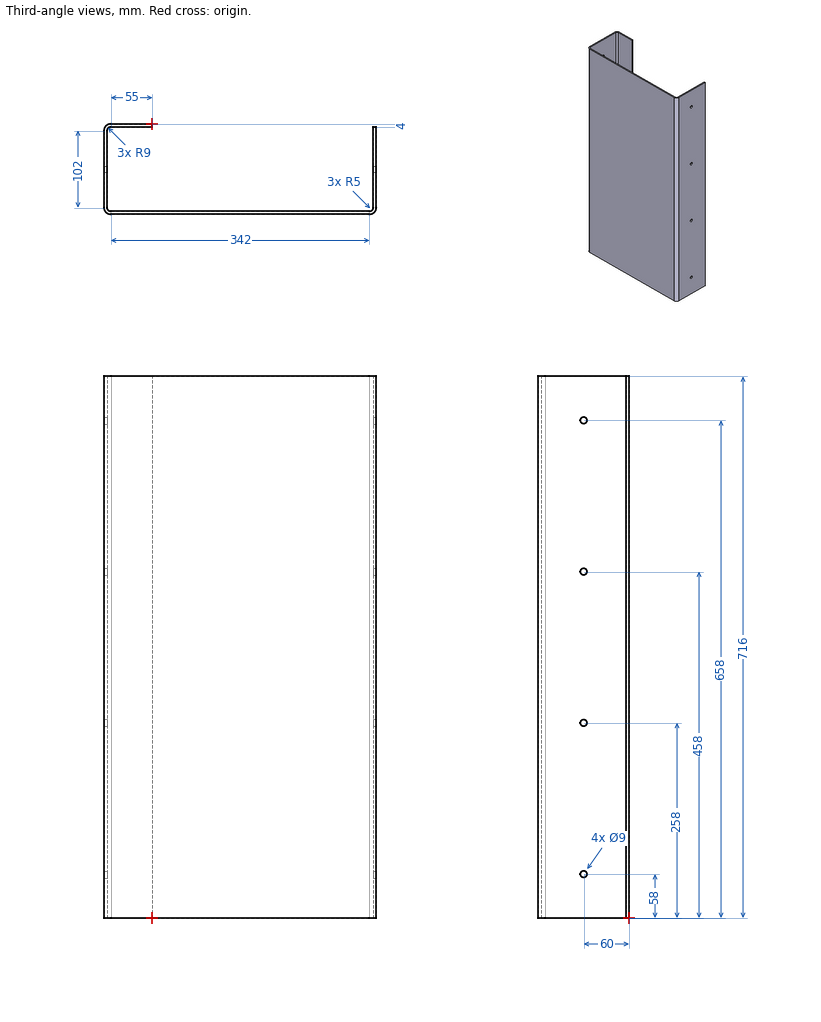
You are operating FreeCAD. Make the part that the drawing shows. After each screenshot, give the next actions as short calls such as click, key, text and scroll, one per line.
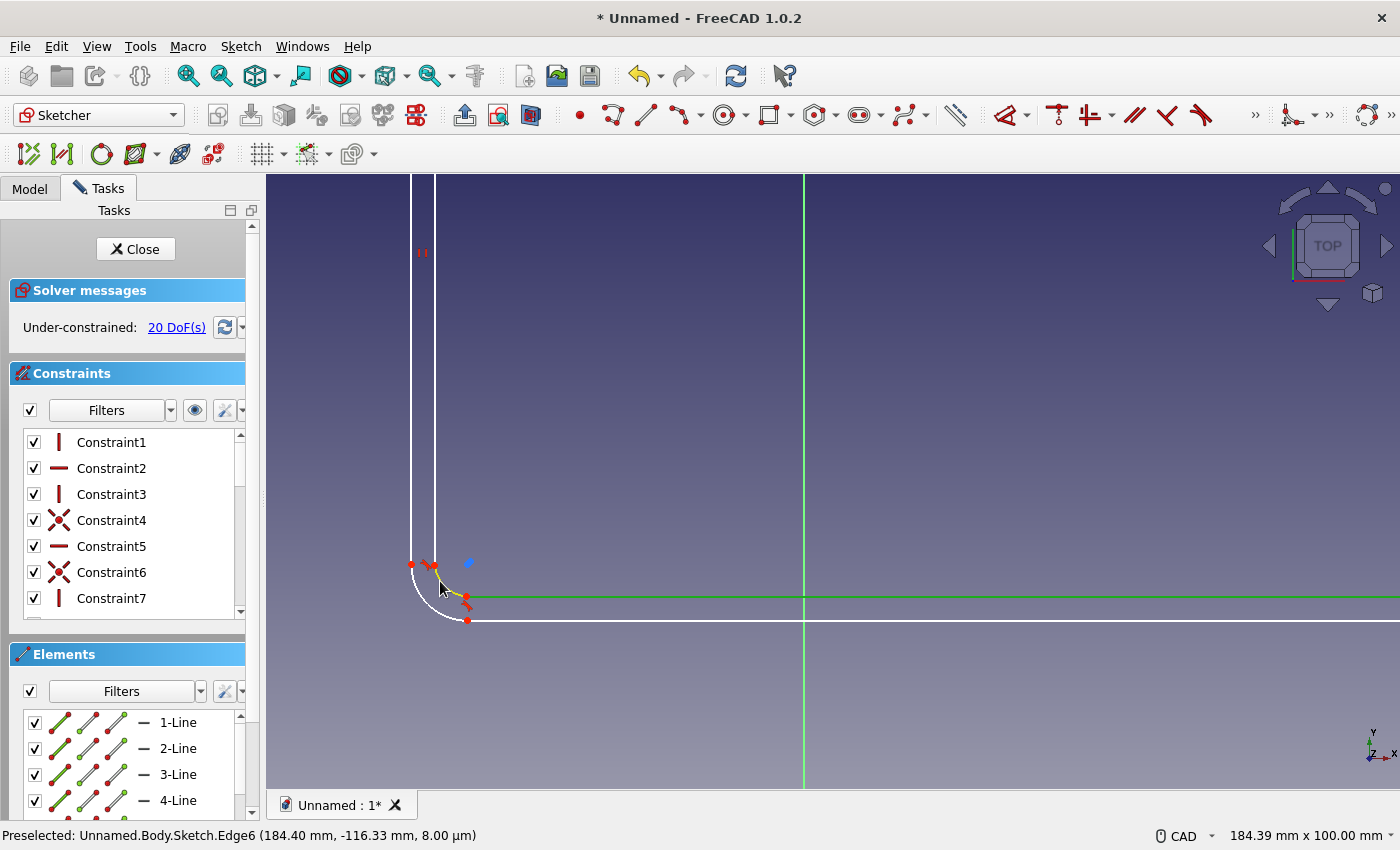
click(439, 579)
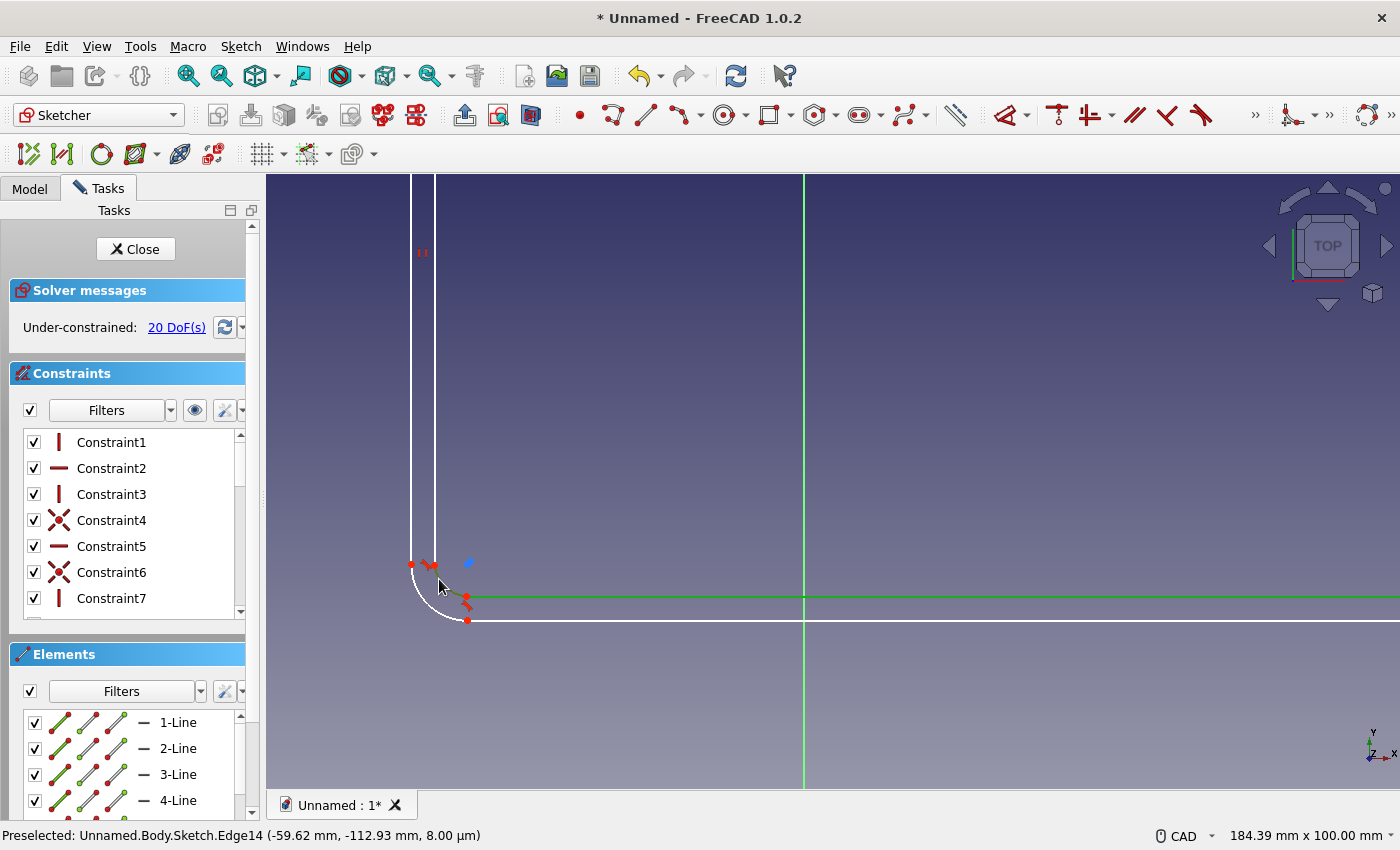
click(1201, 116)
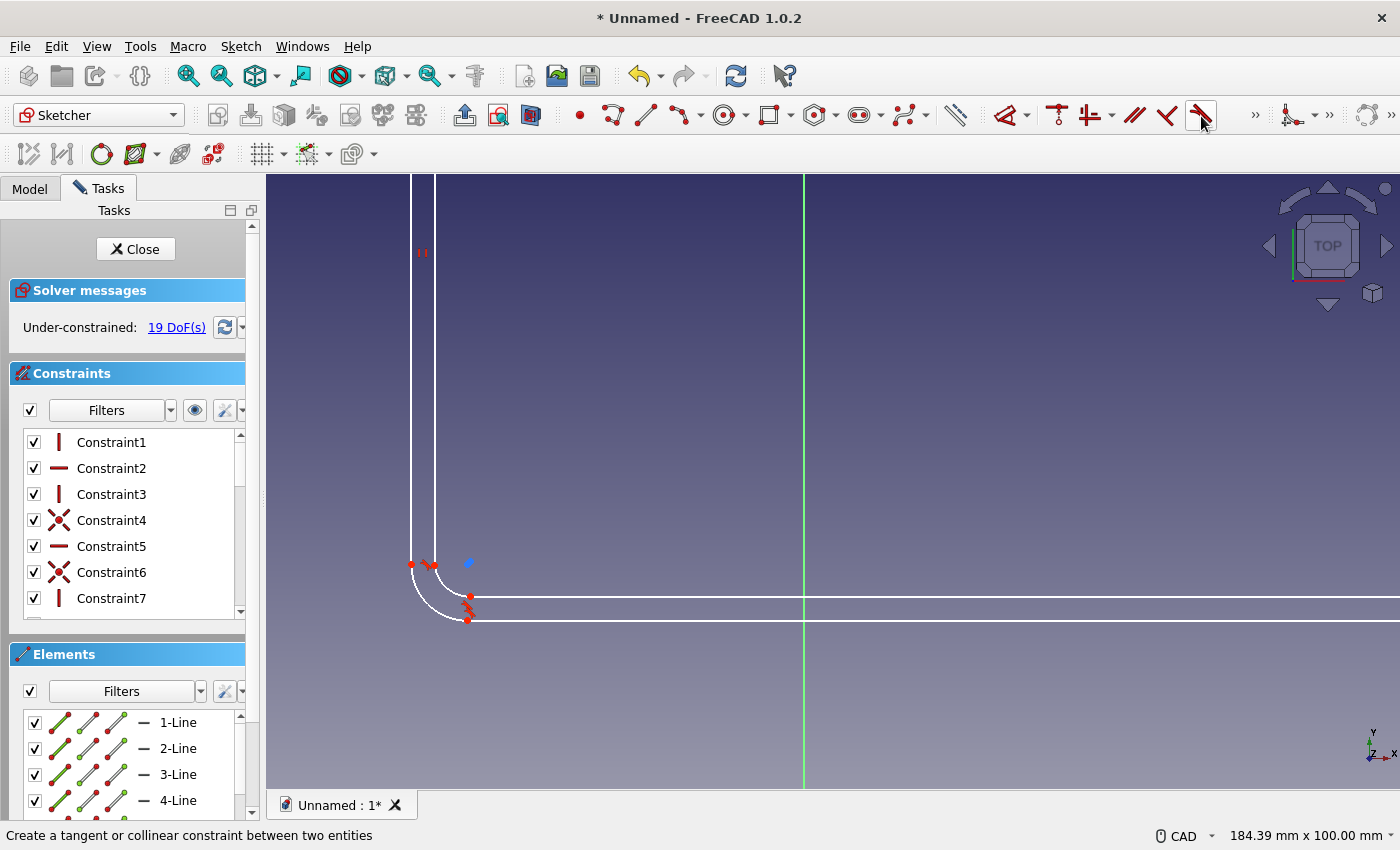
click(435, 378)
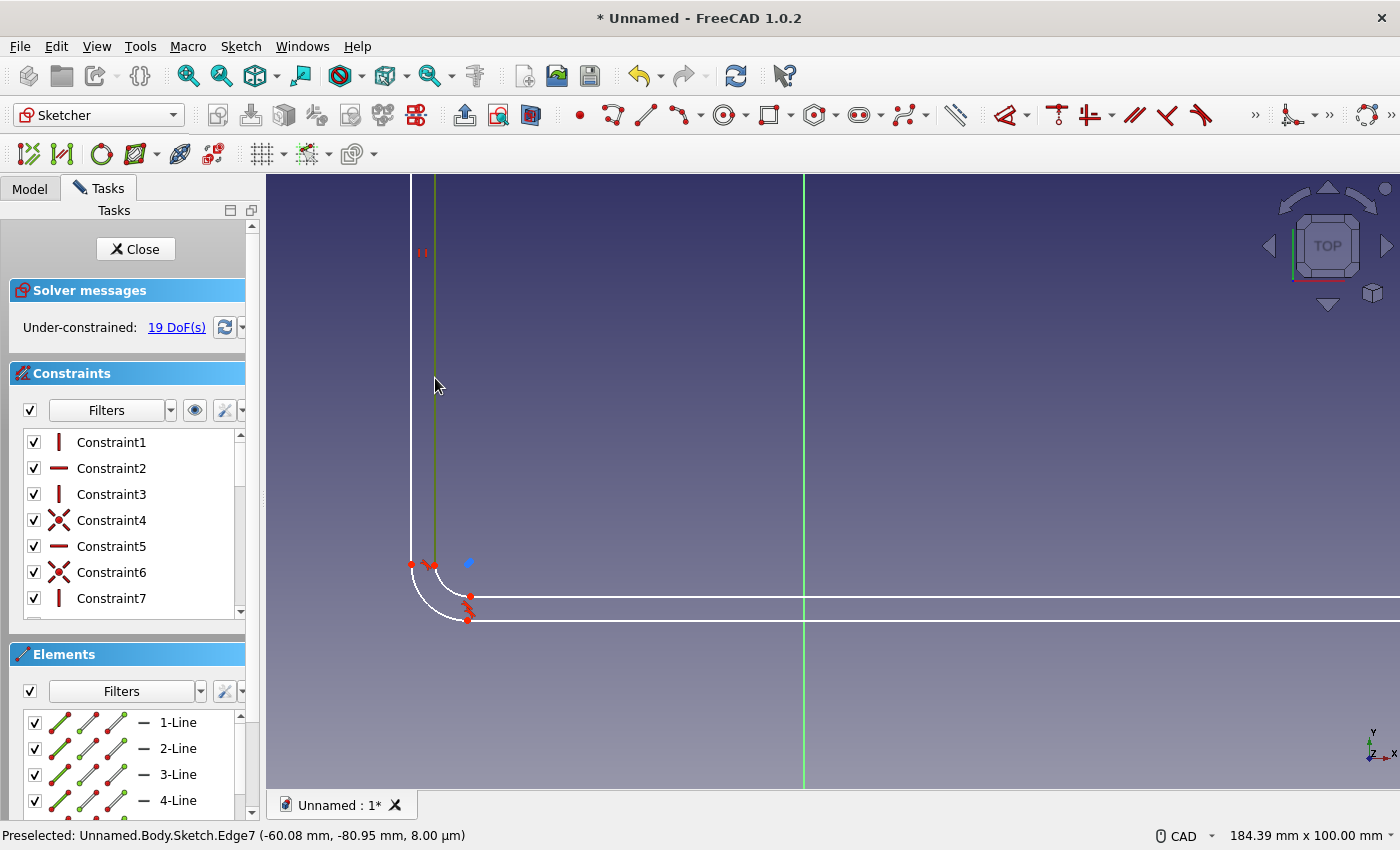
click(440, 580)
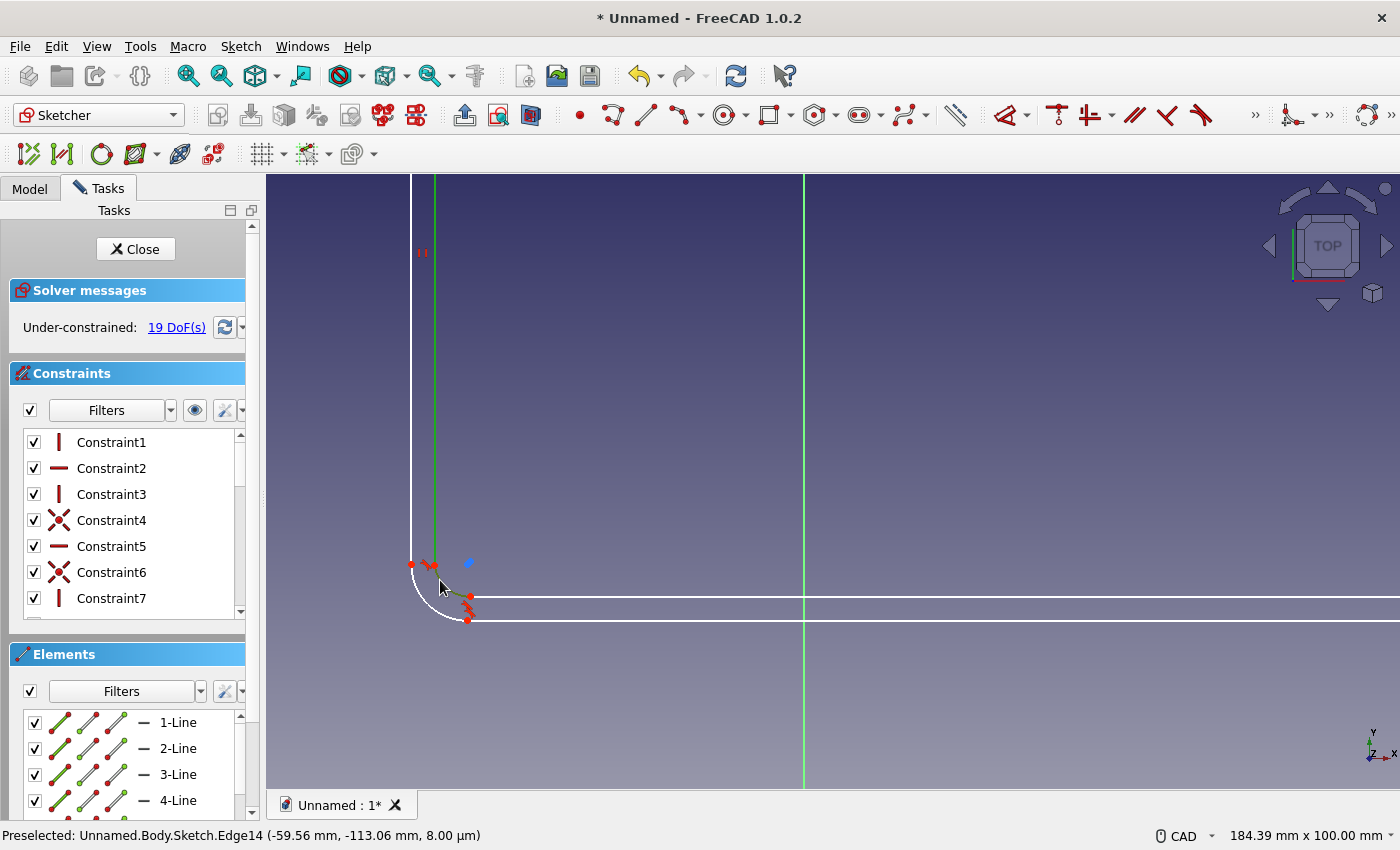
click(1201, 116)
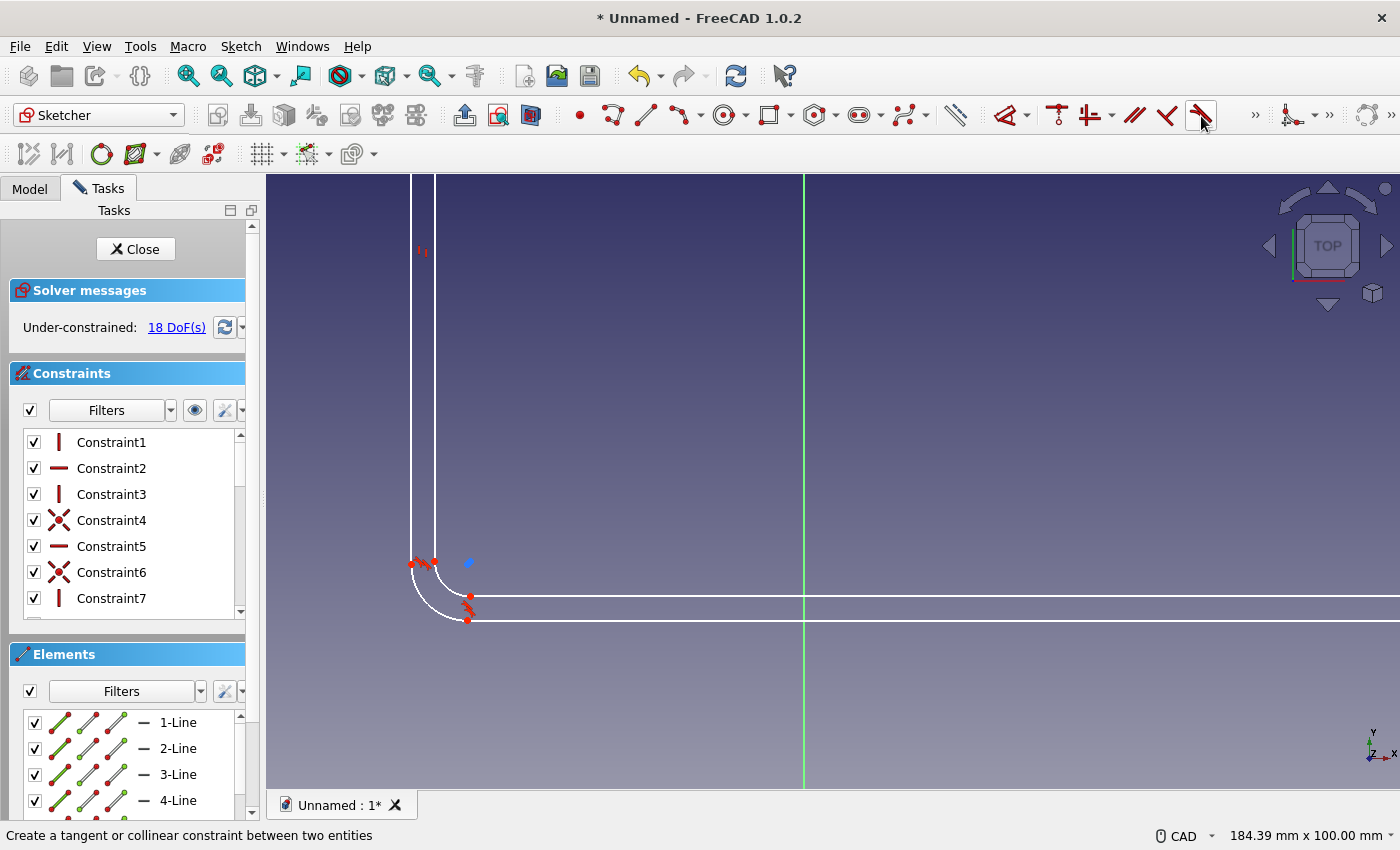
click(435, 374)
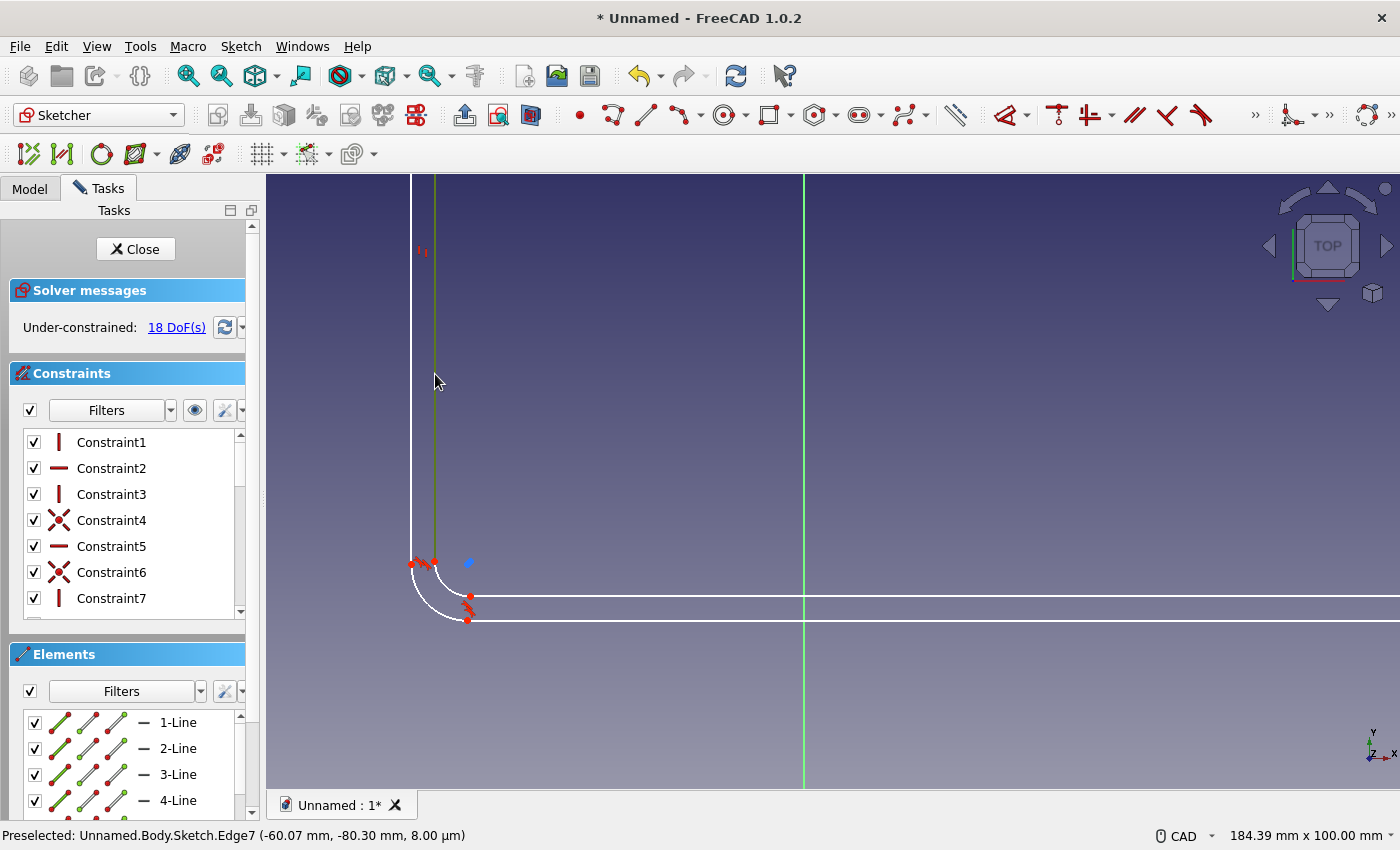
scroll(440, 581, down, 6)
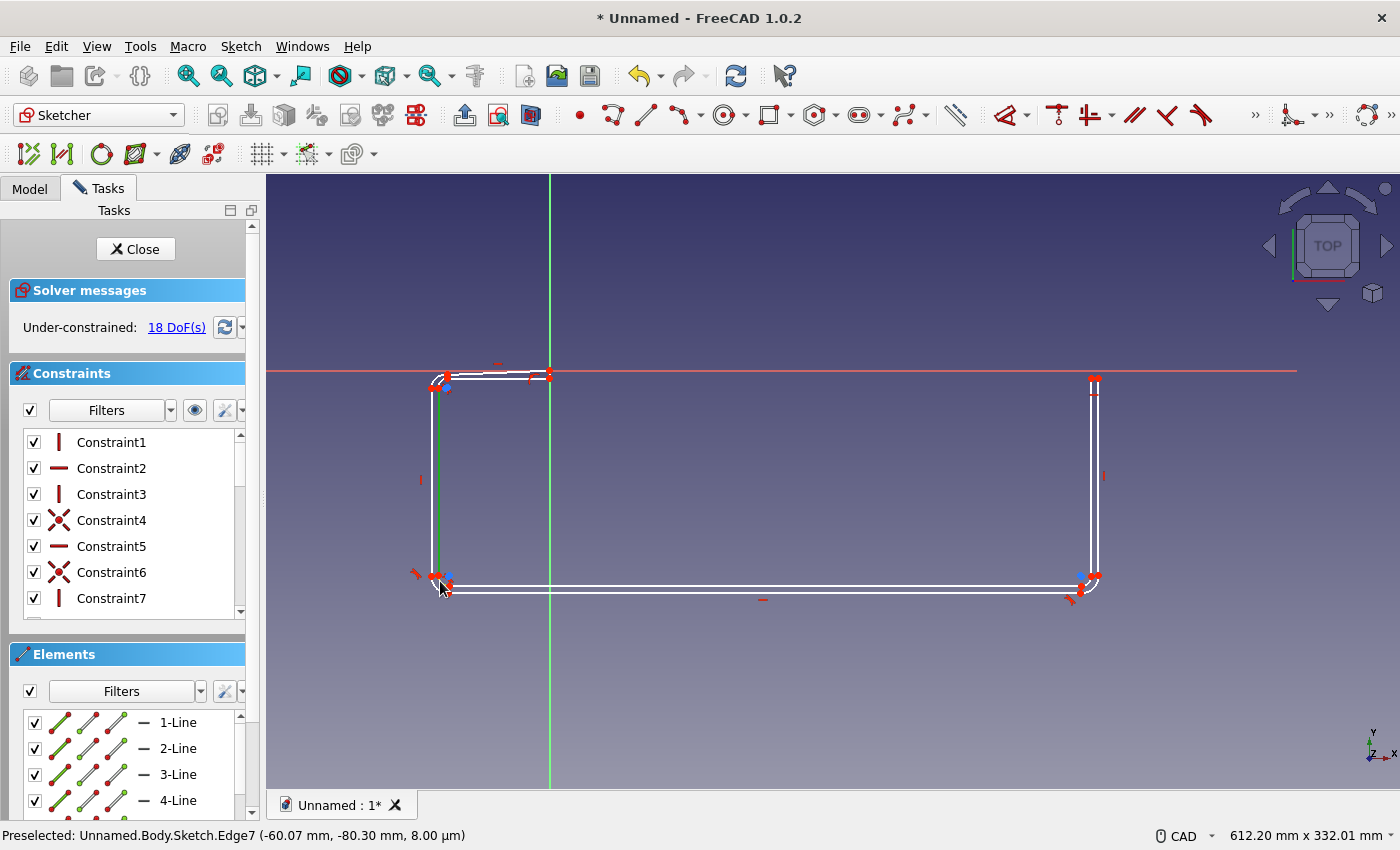
scroll(444, 379, up, 6)